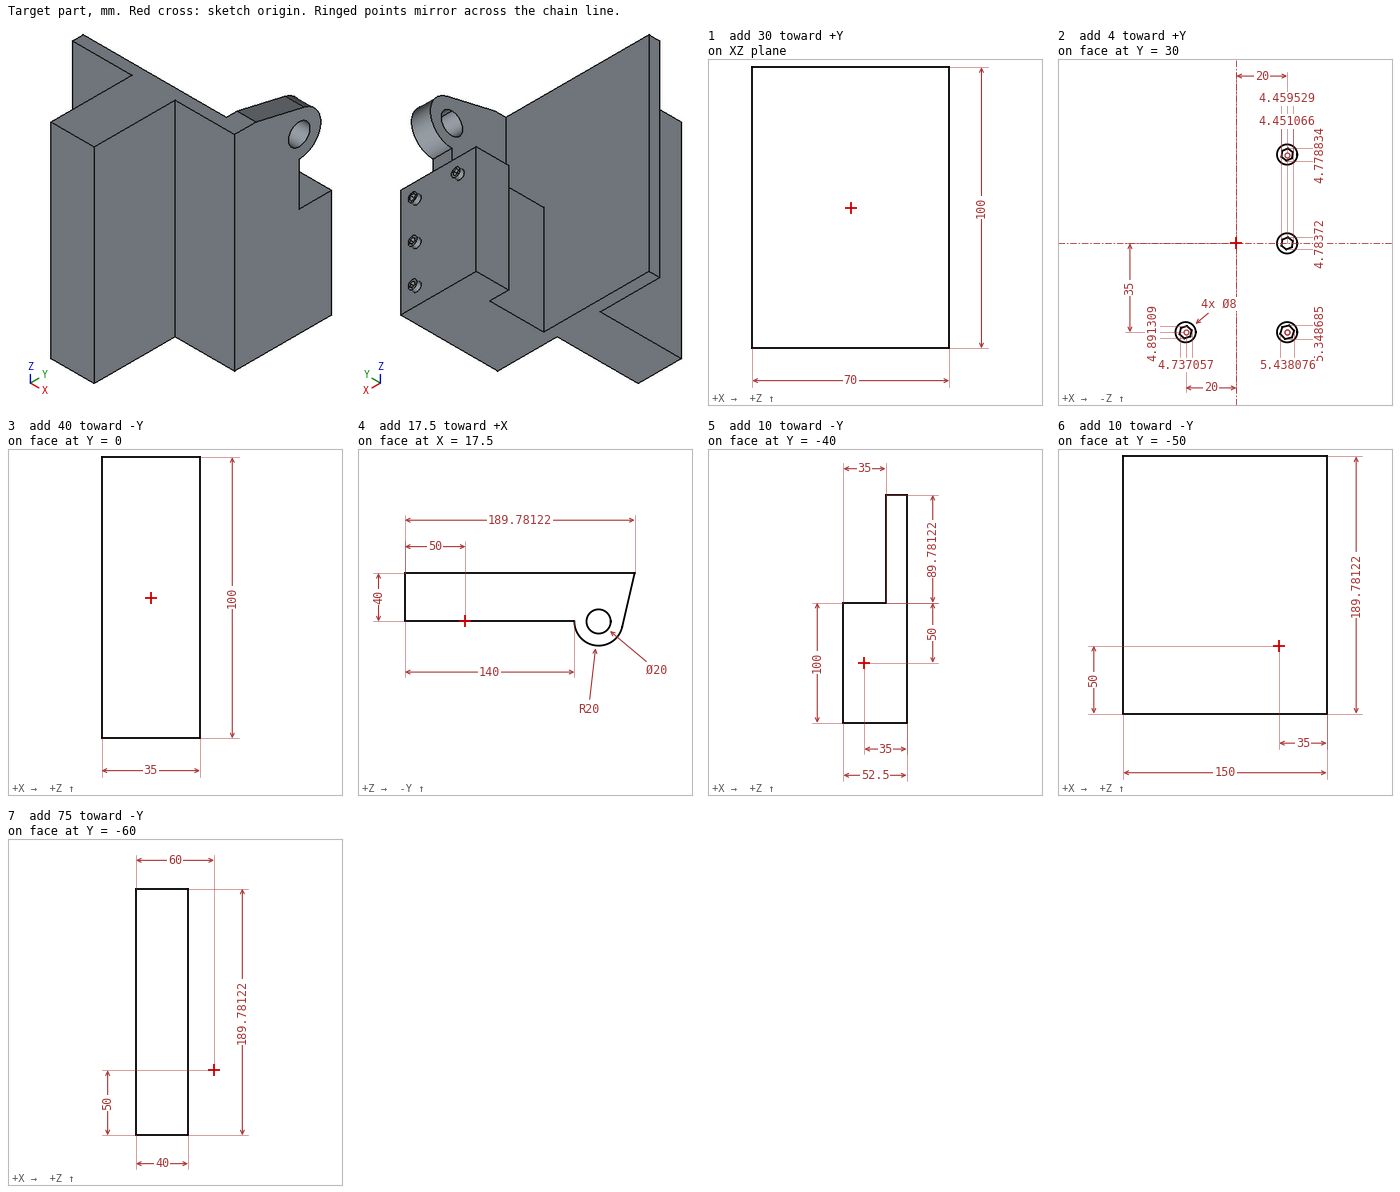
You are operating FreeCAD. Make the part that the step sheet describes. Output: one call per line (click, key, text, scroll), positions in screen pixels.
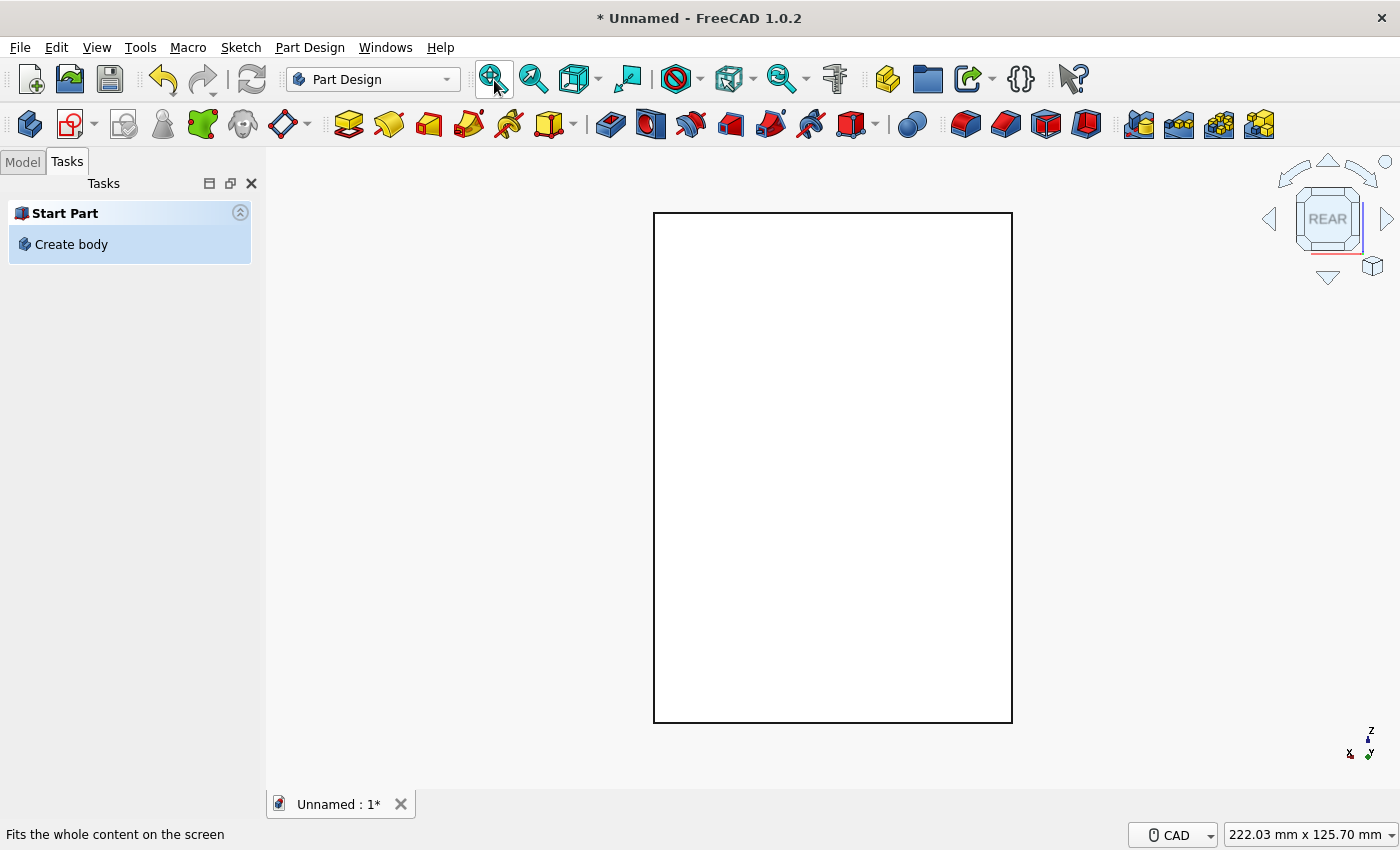
click(833, 394)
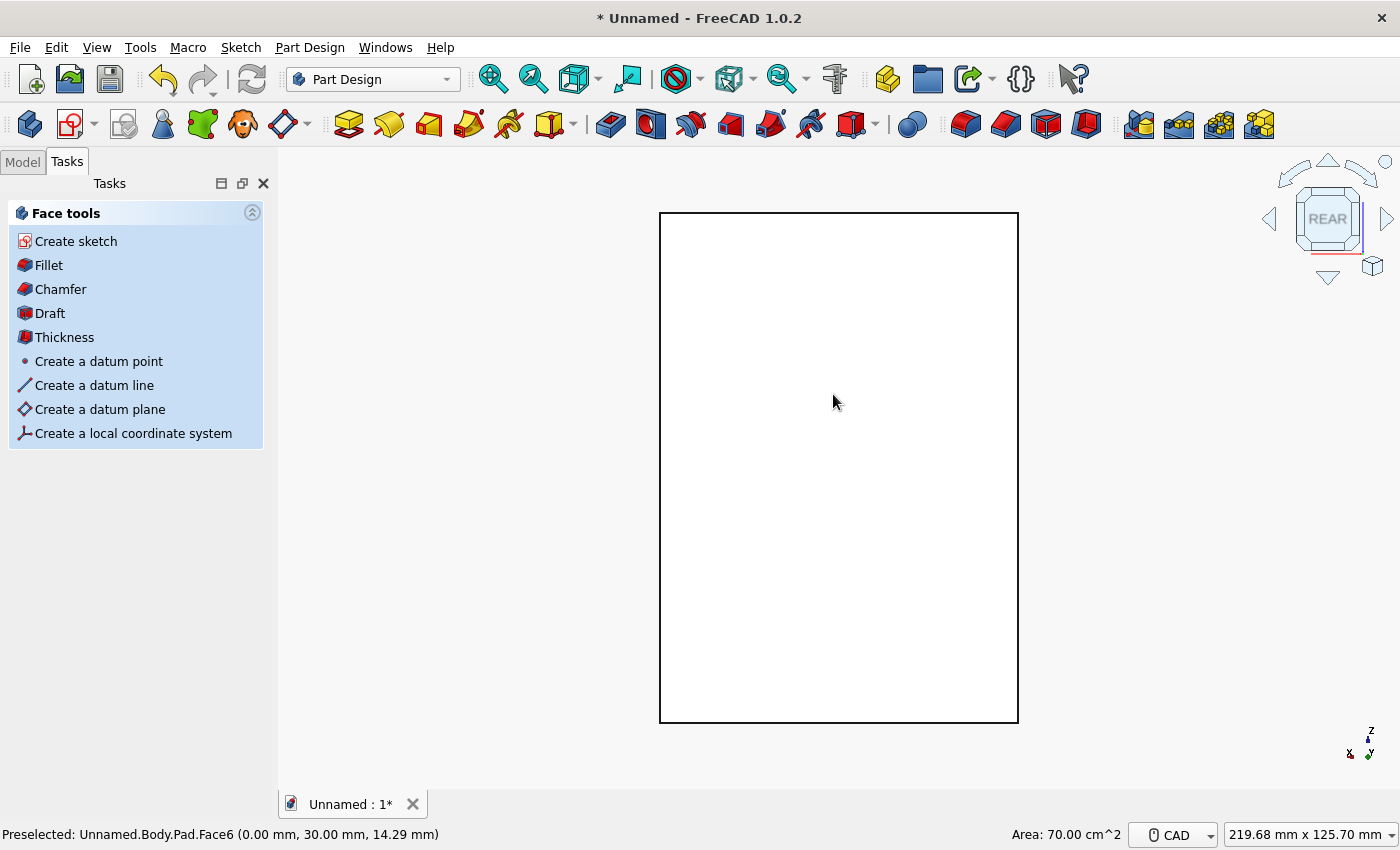
click(70, 124)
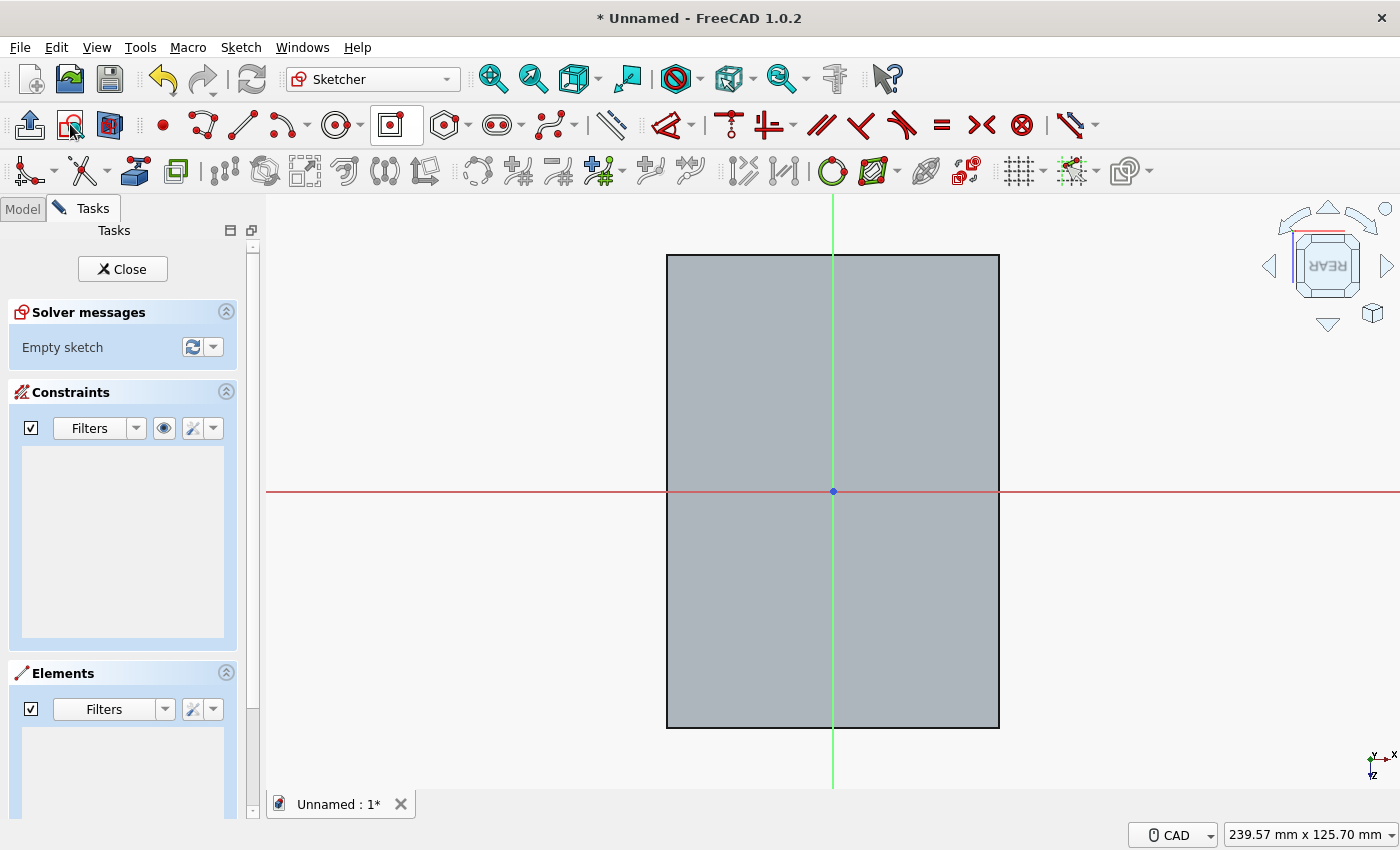
key(g)
key(p)
key(6)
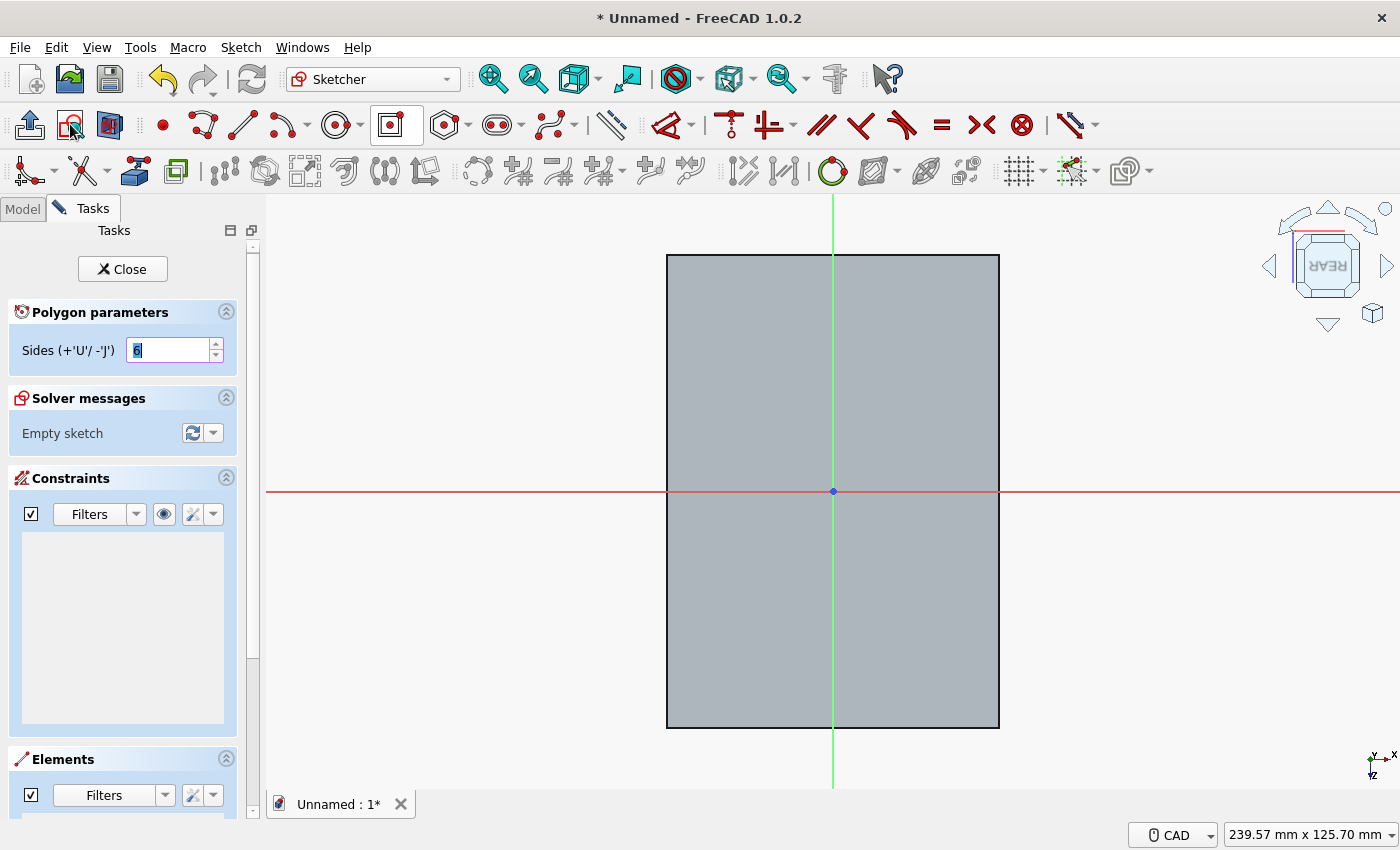
scroll(738, 657, up, 5)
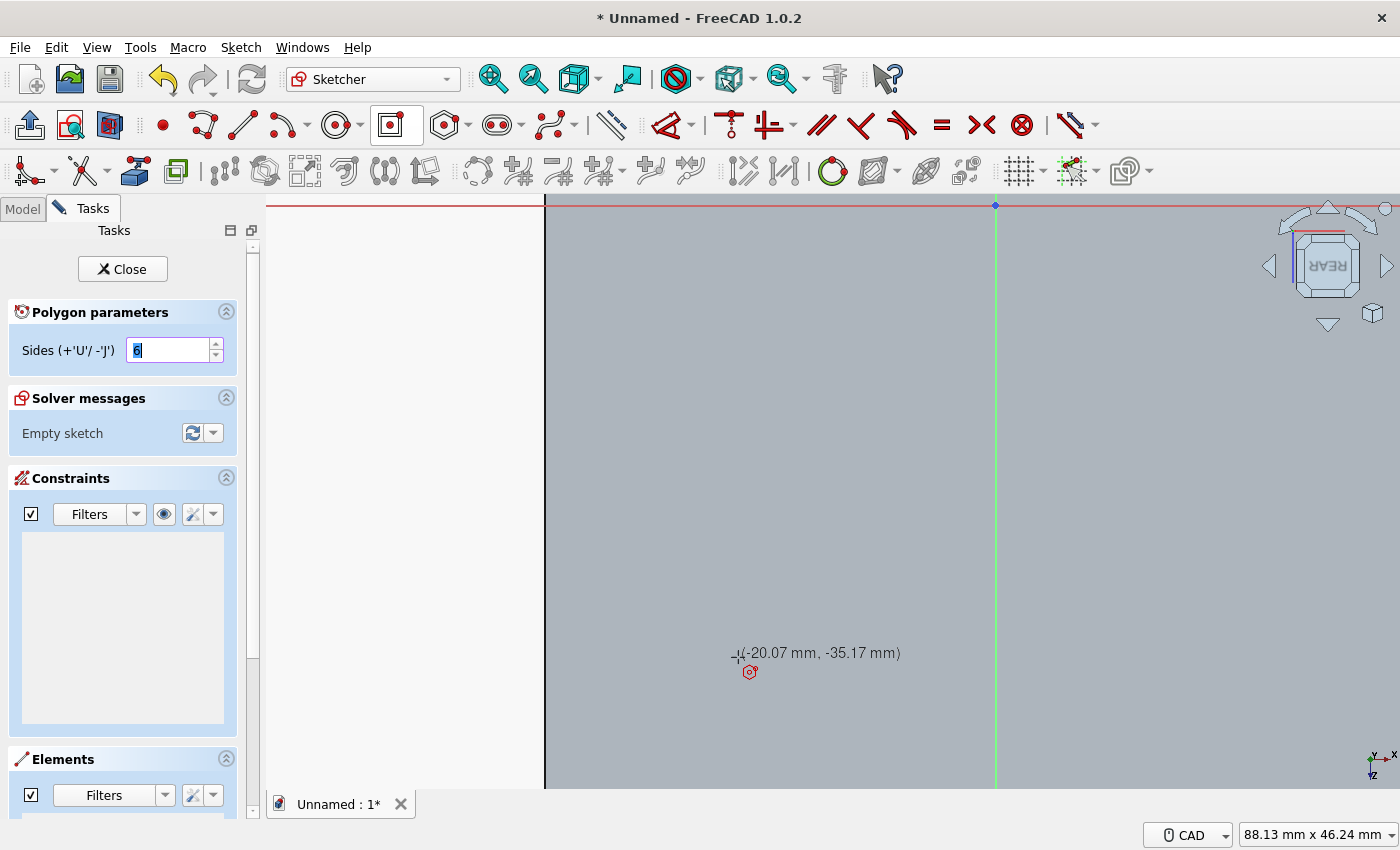
click(738, 656)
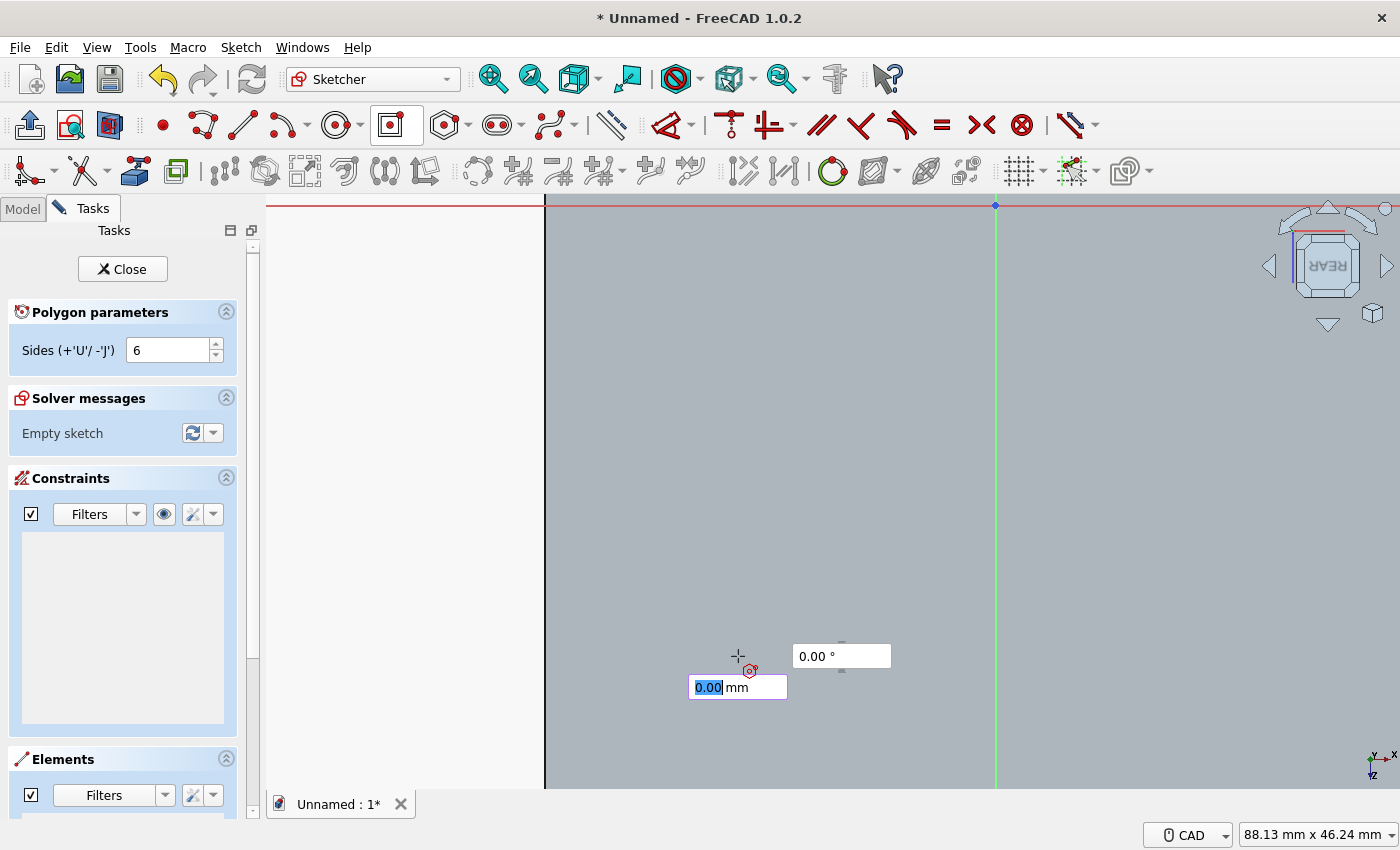
click(708, 666)
right_click(708, 666)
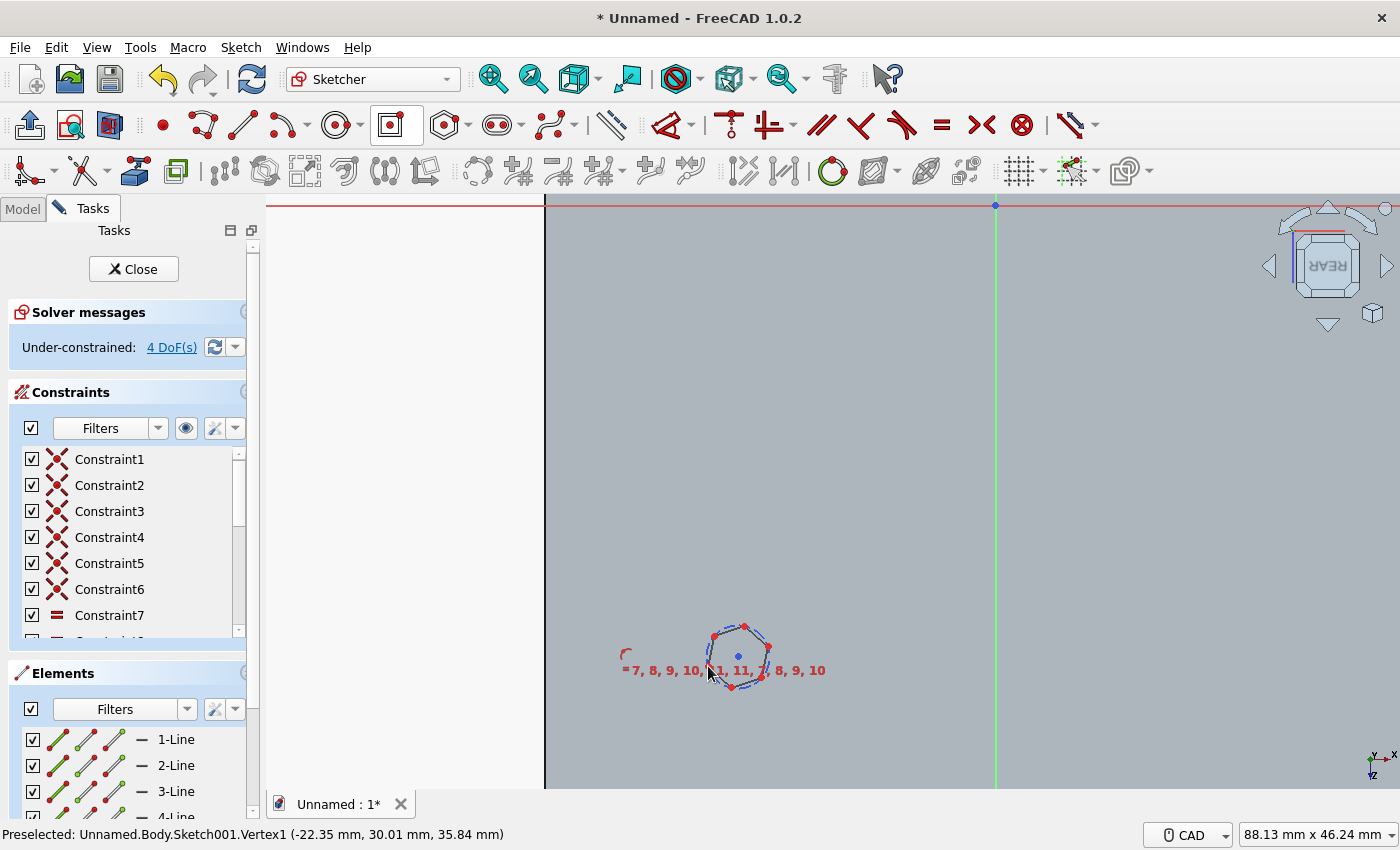
click(444, 126)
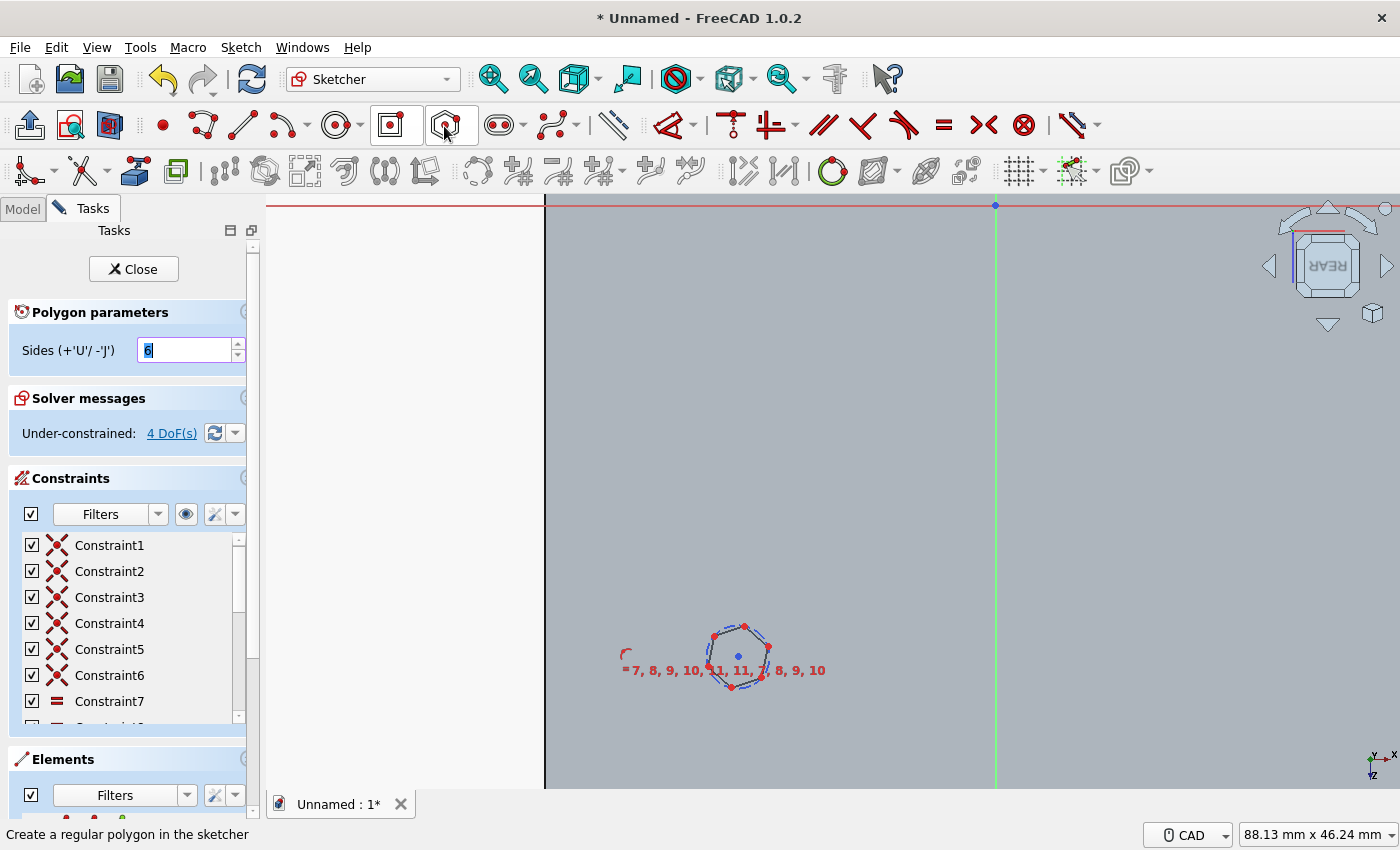
scroll(630, 658, down, 5)